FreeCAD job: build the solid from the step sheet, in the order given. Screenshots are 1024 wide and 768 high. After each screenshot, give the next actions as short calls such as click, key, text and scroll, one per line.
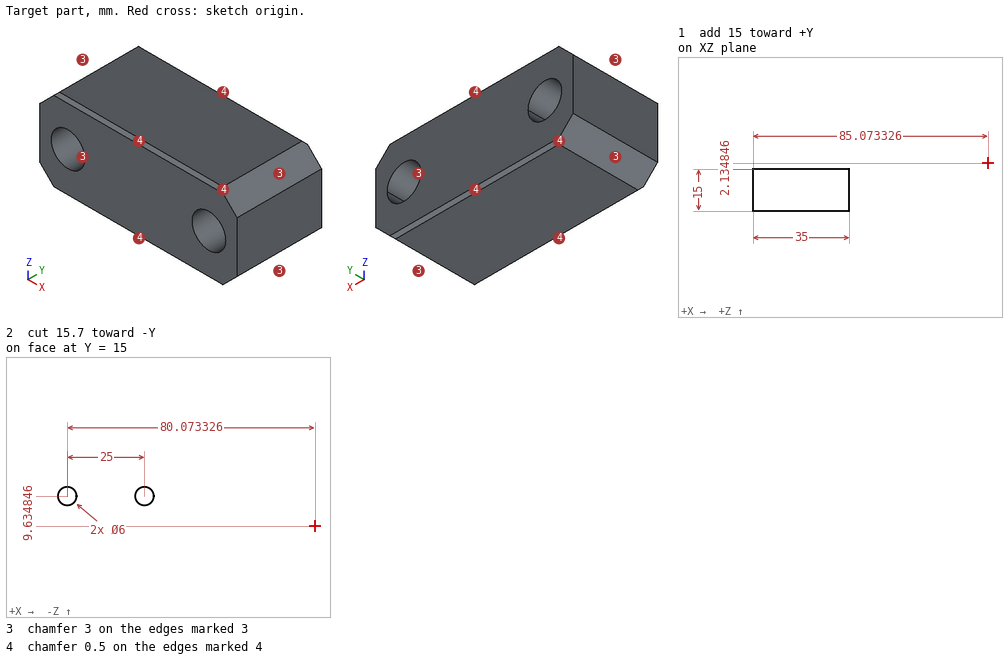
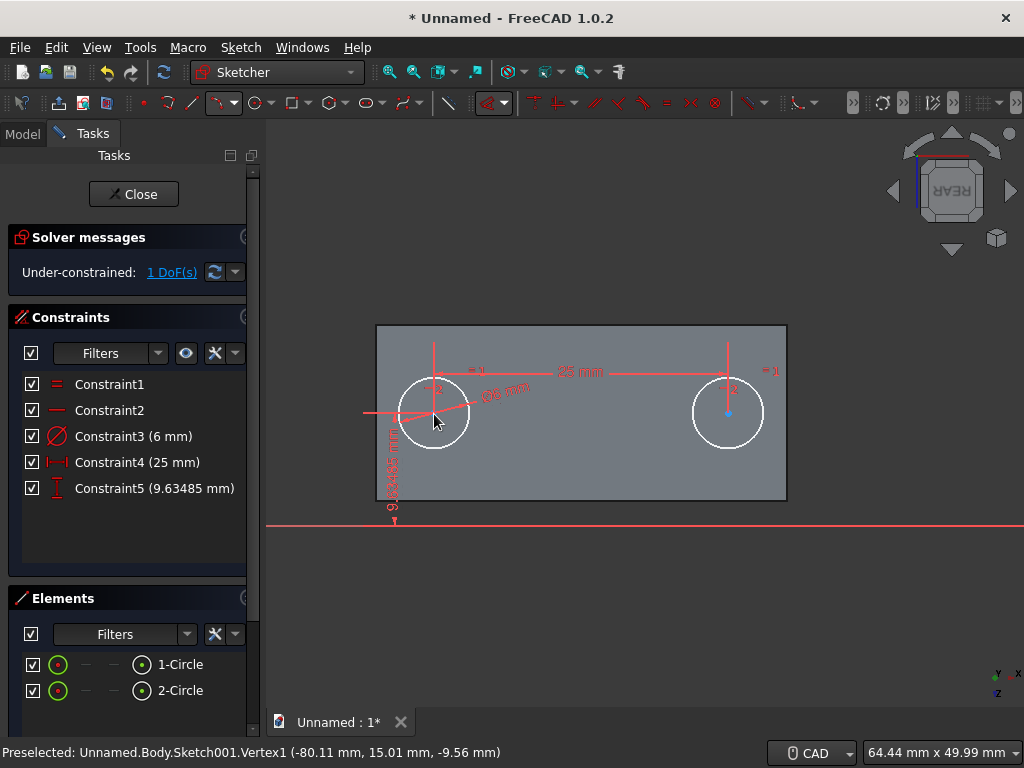
click(434, 413)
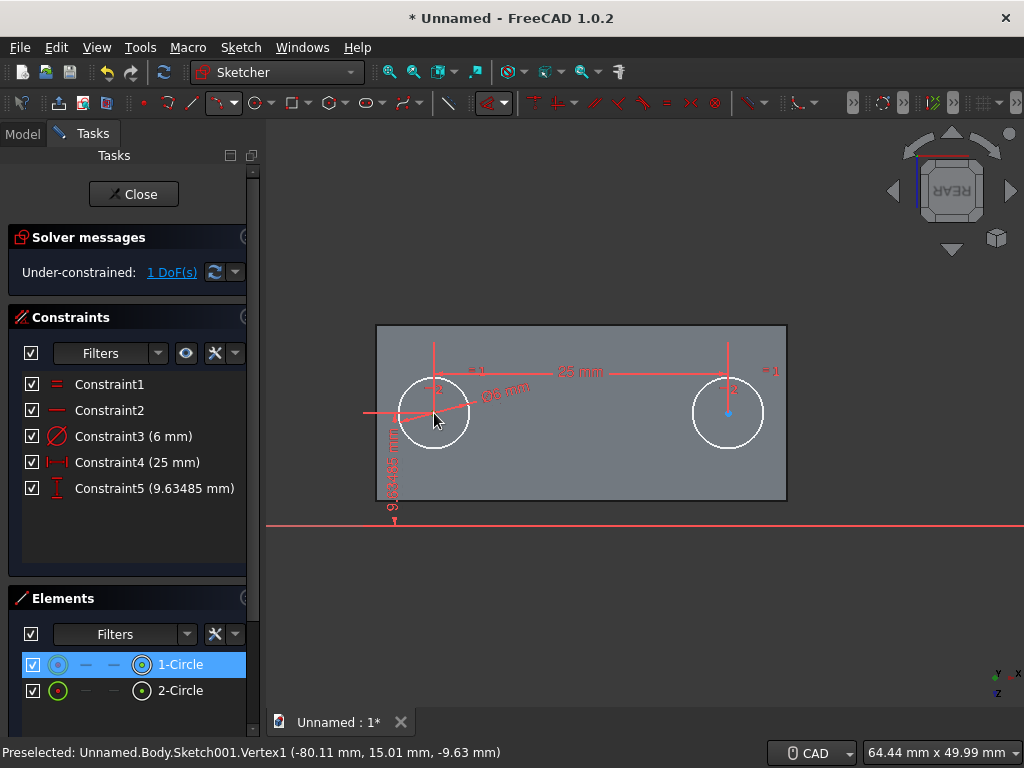
key(l)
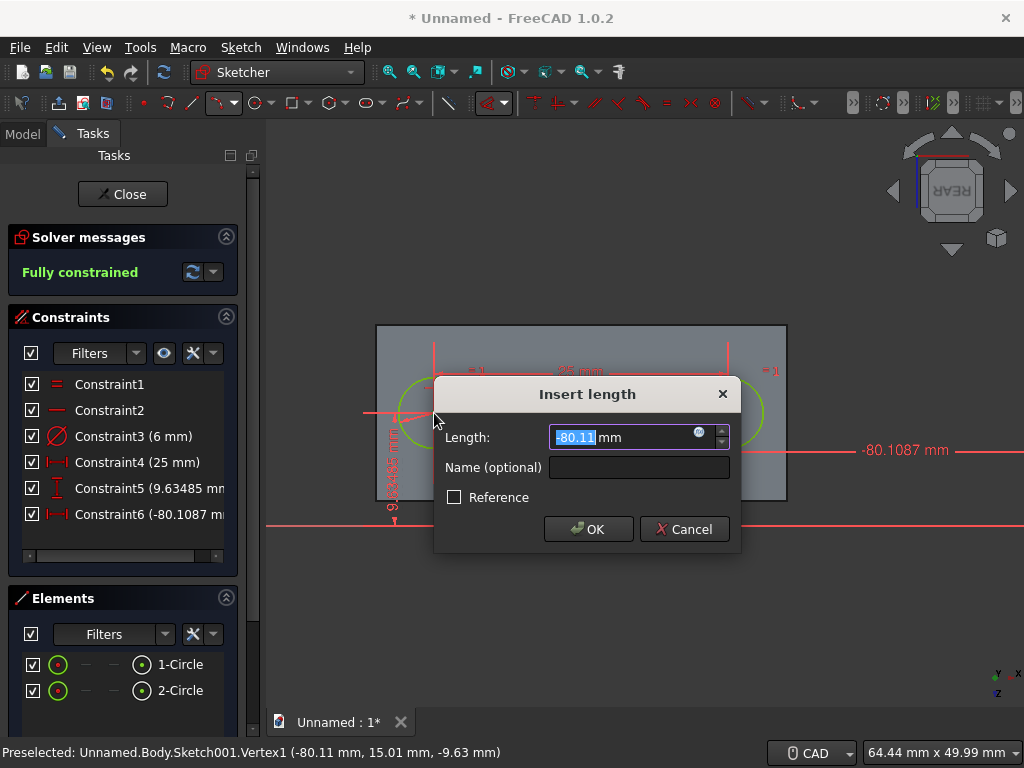
text(-80.073326)
key(Return)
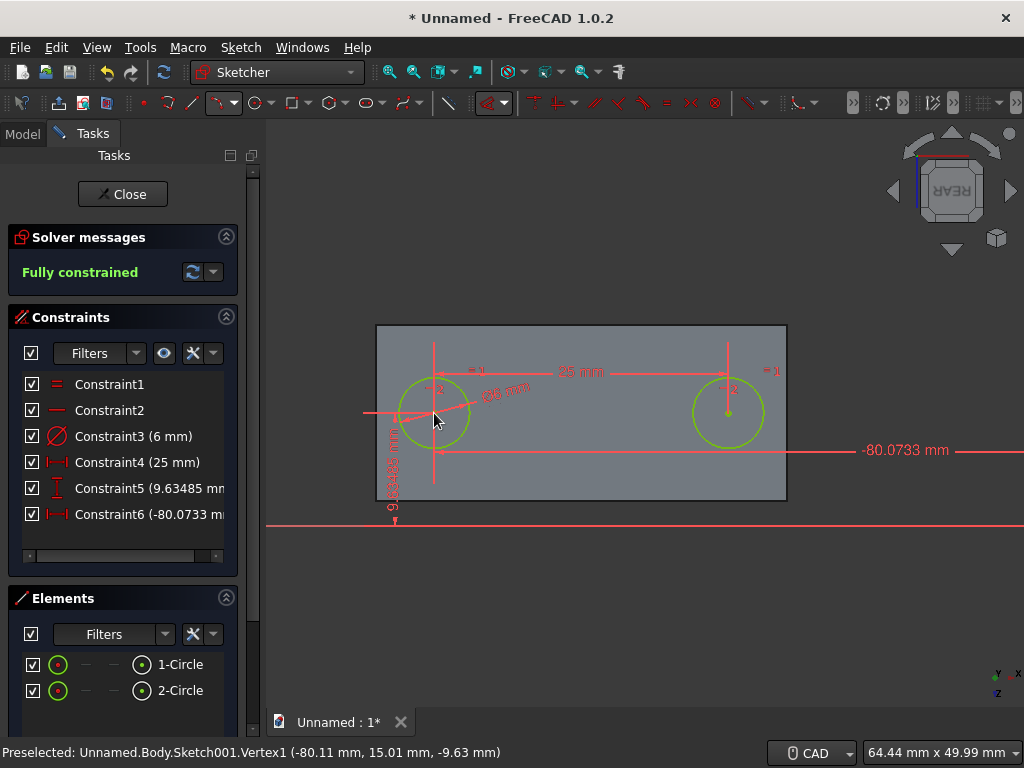
click(123, 194)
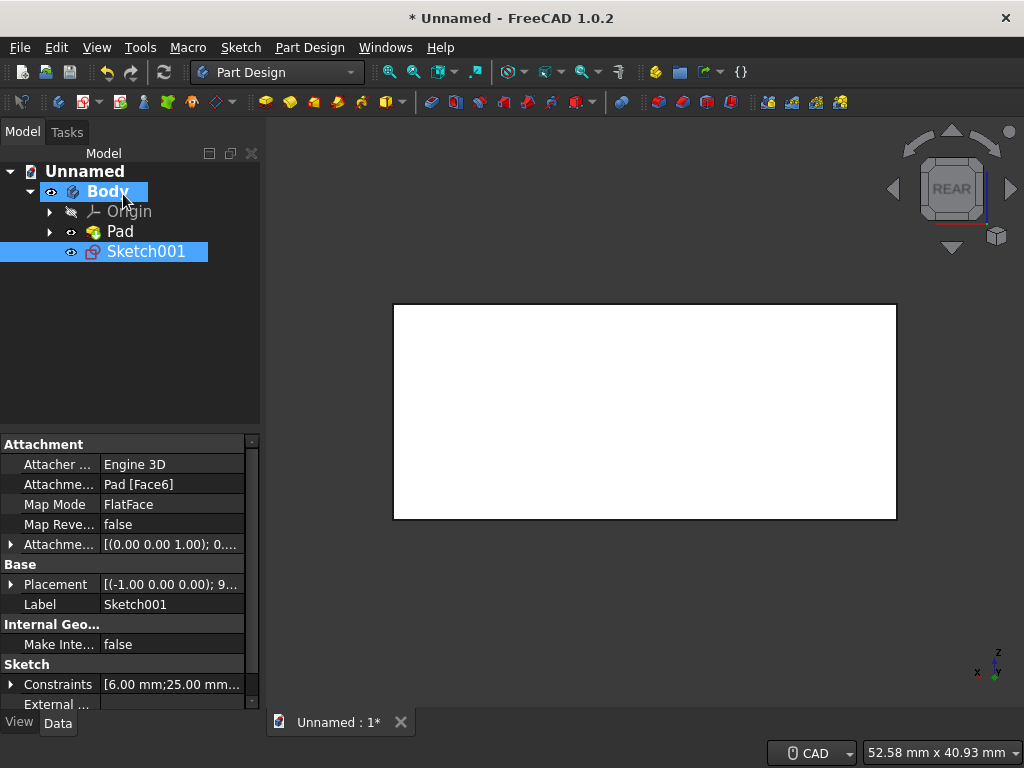
click(432, 102)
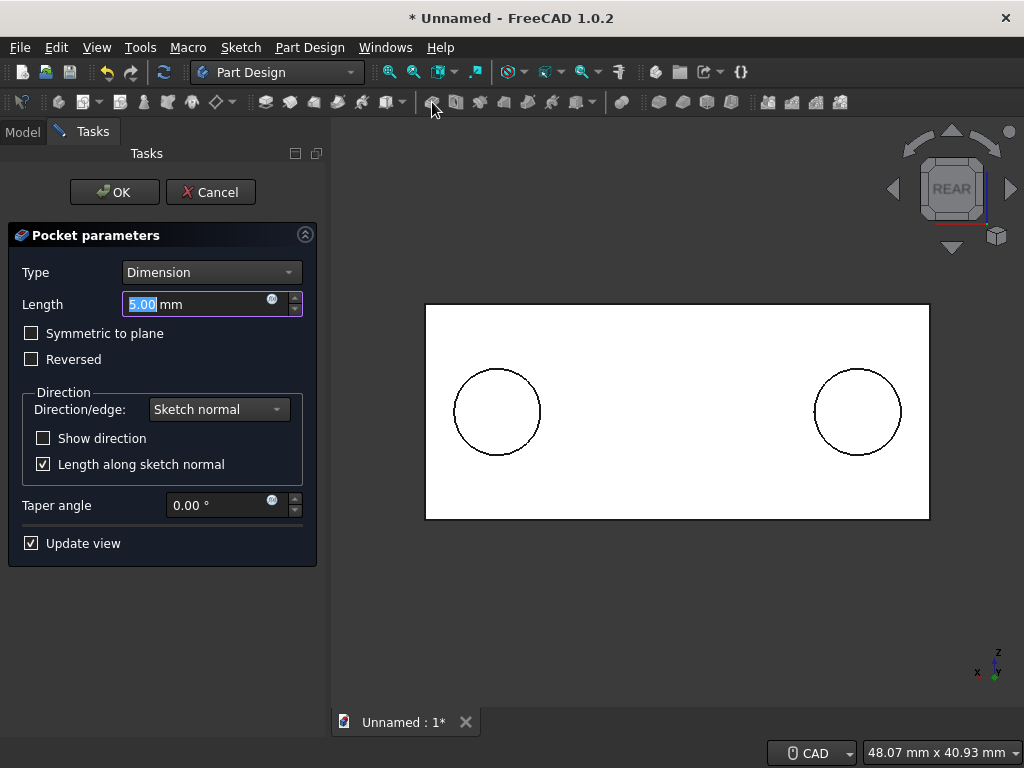
text(15.7)
key(Tab)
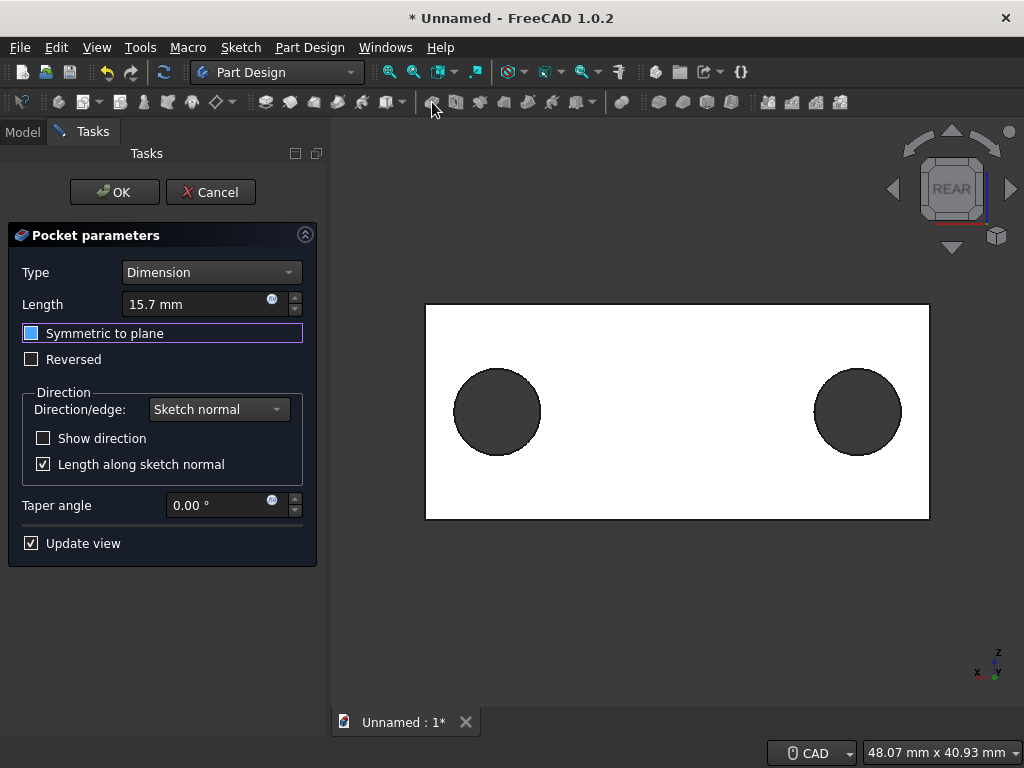
click(115, 192)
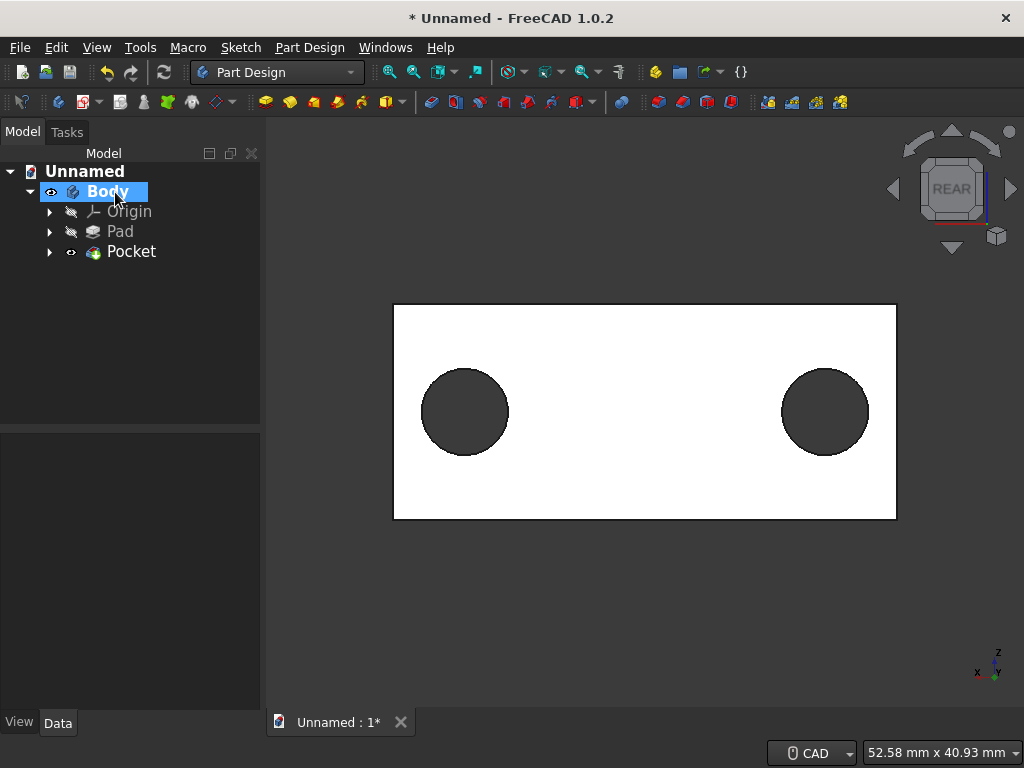
key(0)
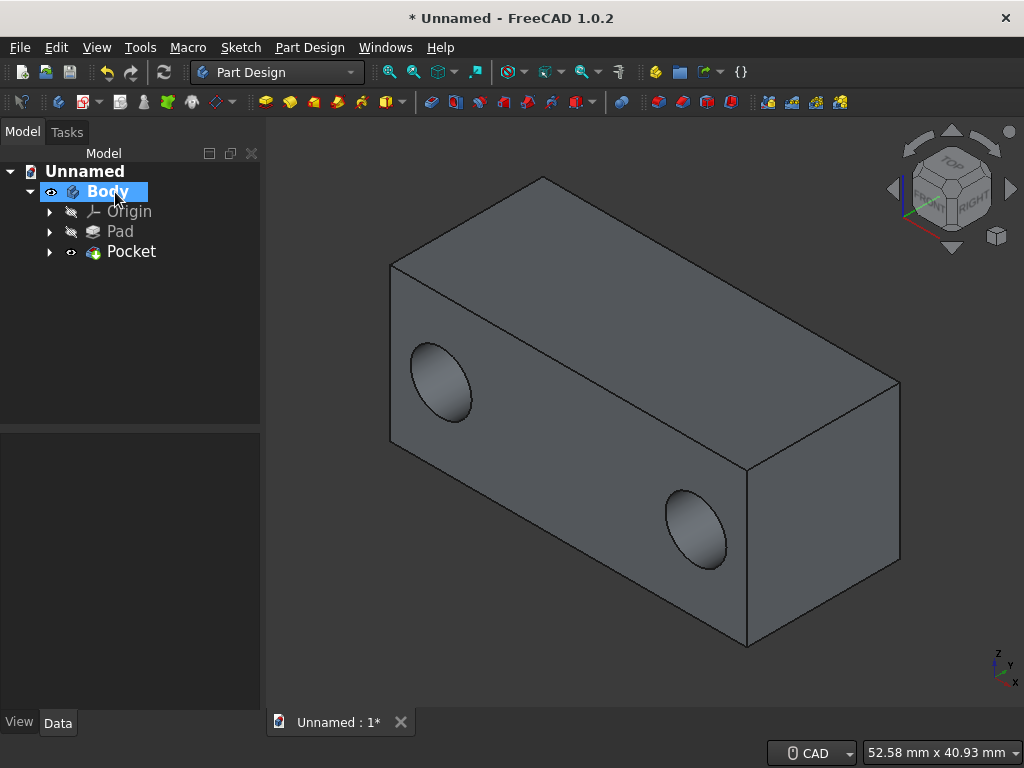
click(823, 426)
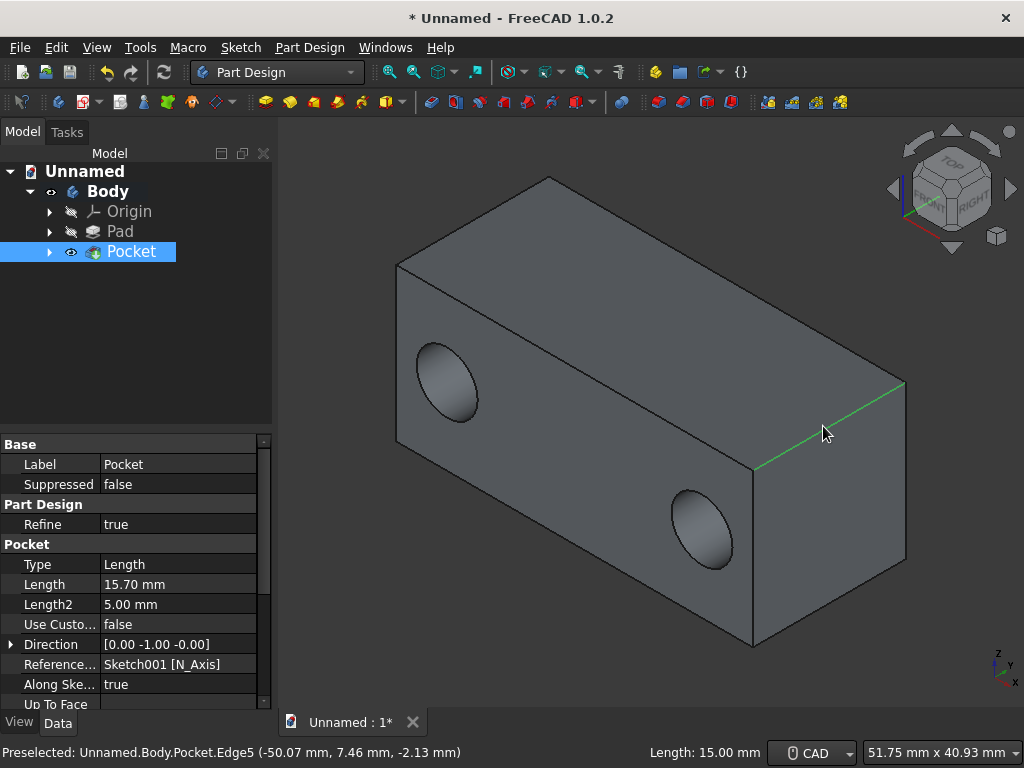
key(2)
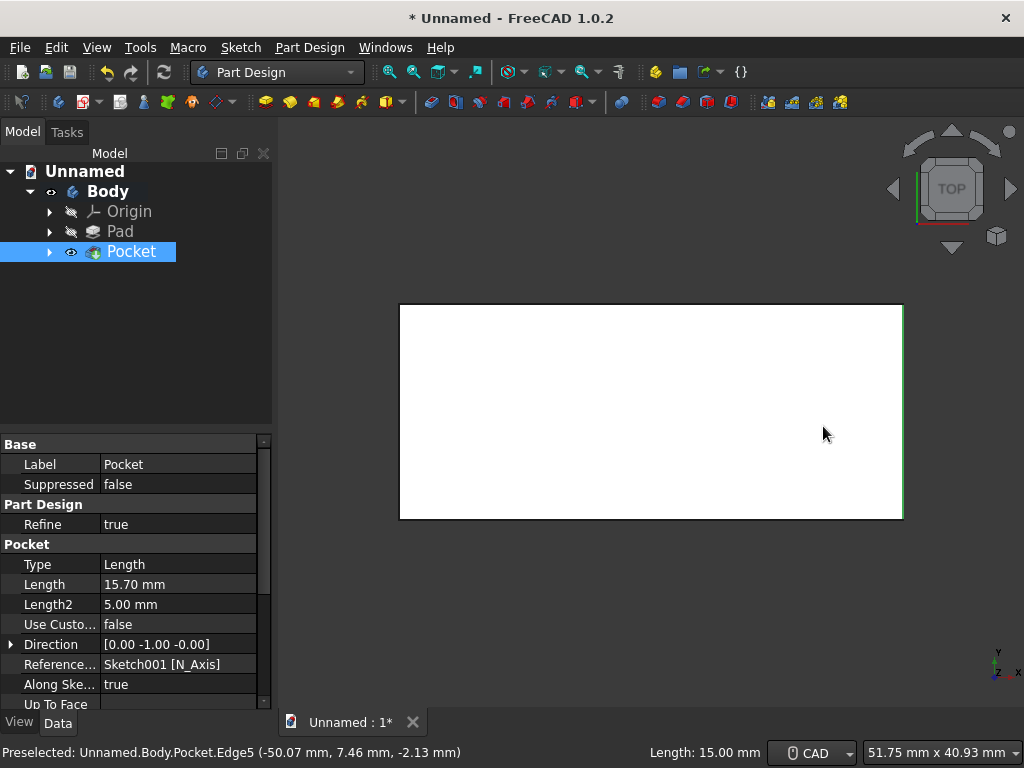
click(399, 411, ctrl)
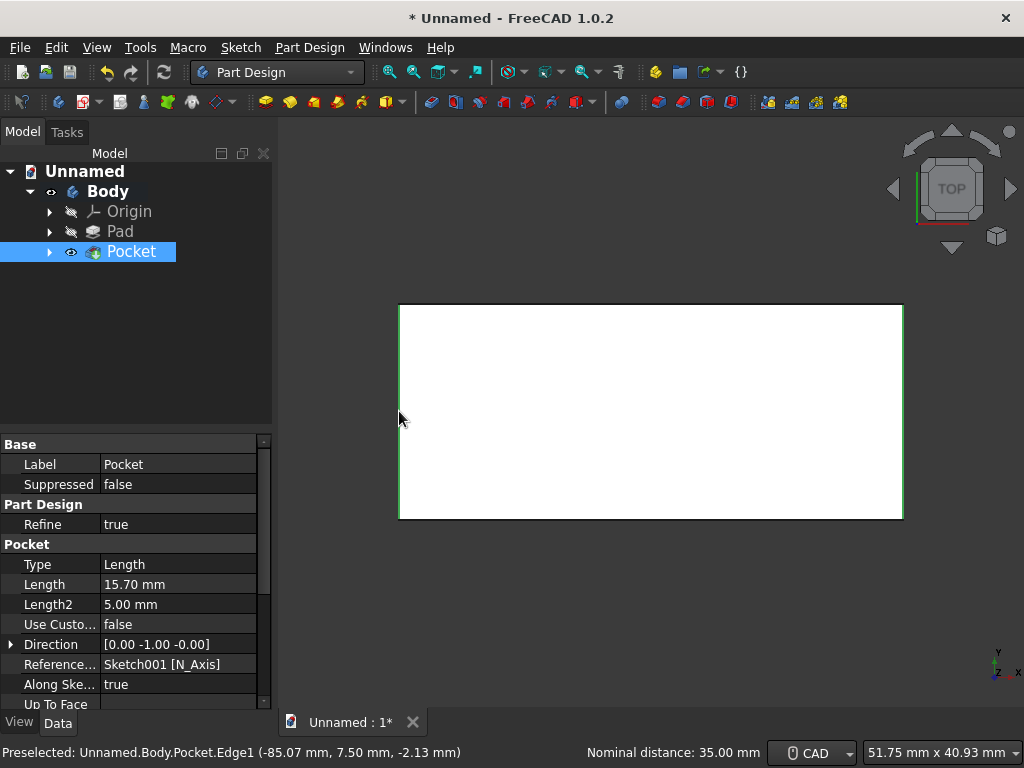
key(1)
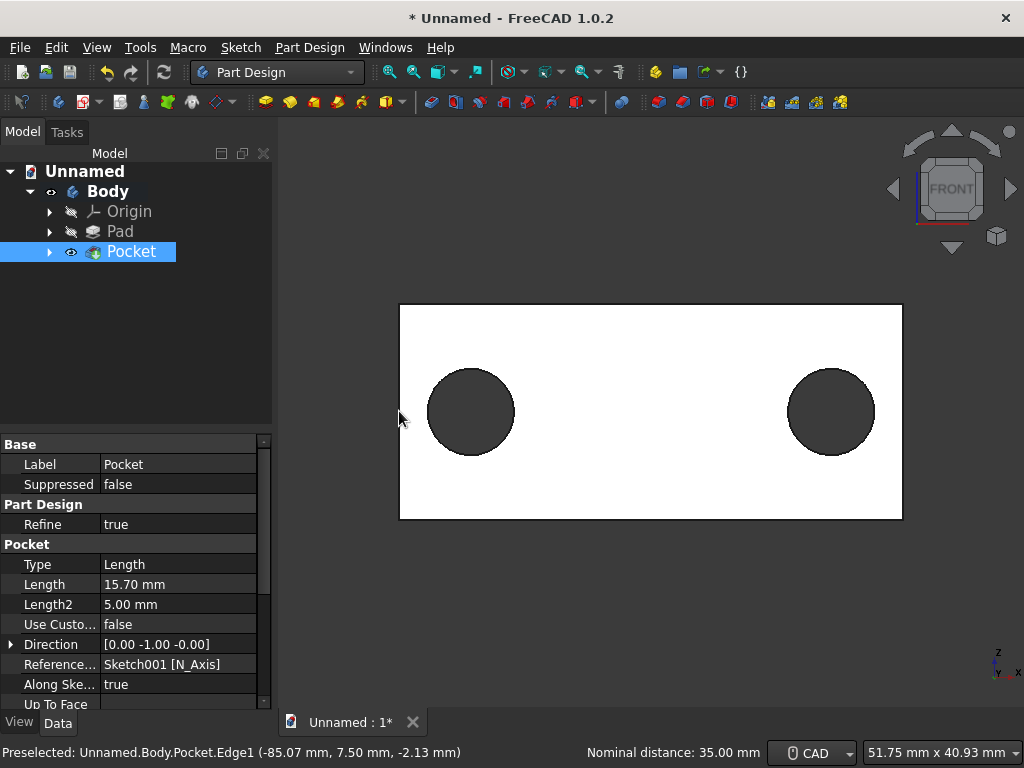
key(3)